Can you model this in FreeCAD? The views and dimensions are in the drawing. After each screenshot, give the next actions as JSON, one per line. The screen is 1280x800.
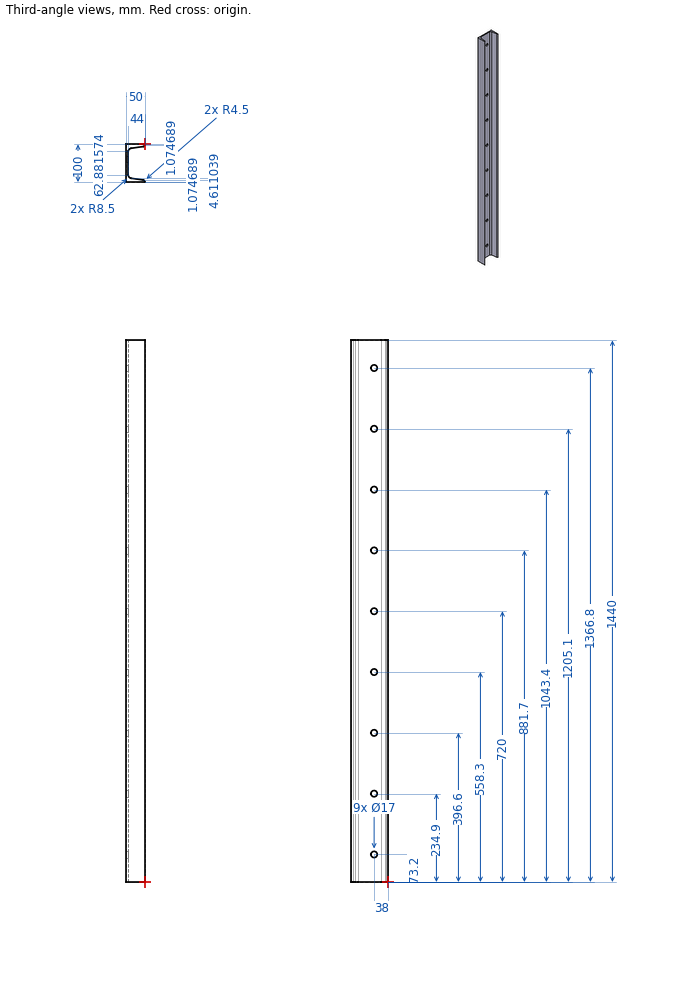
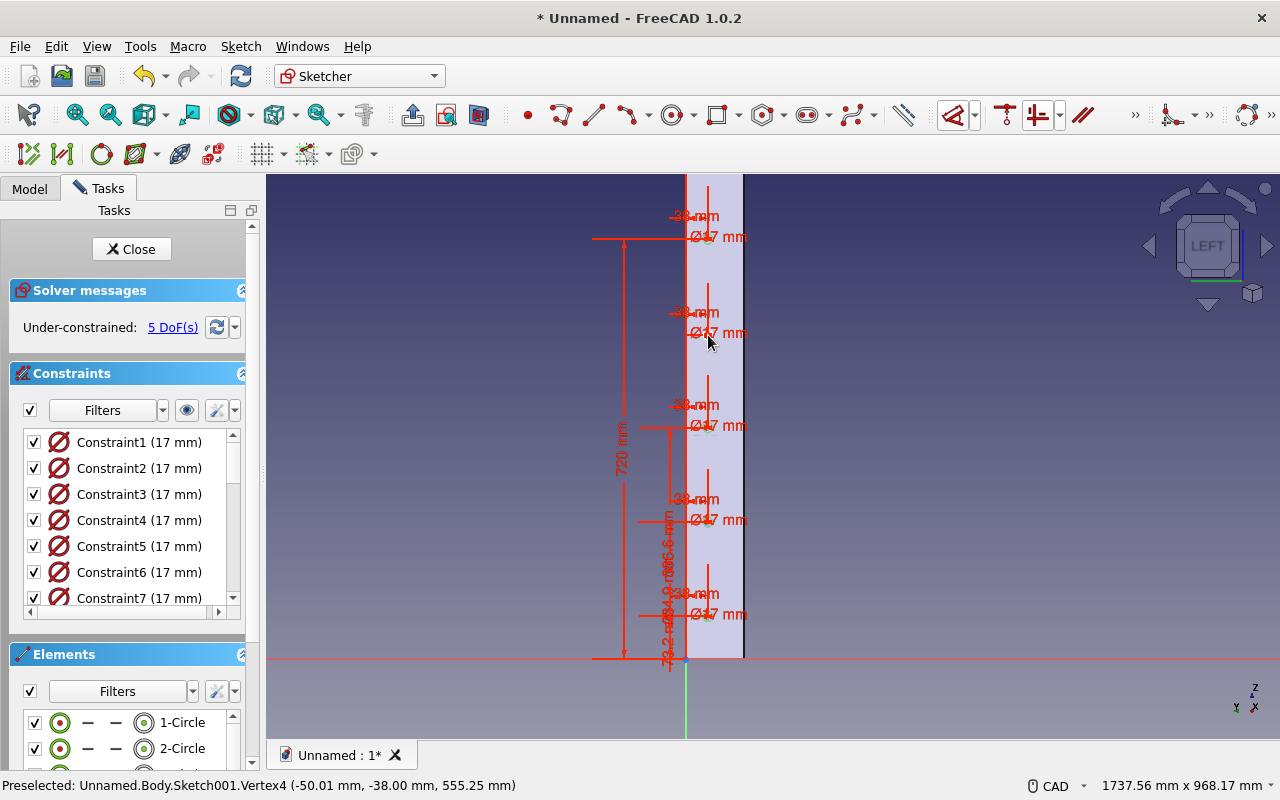
{"action": "left_click", "coordinate": [974, 116]}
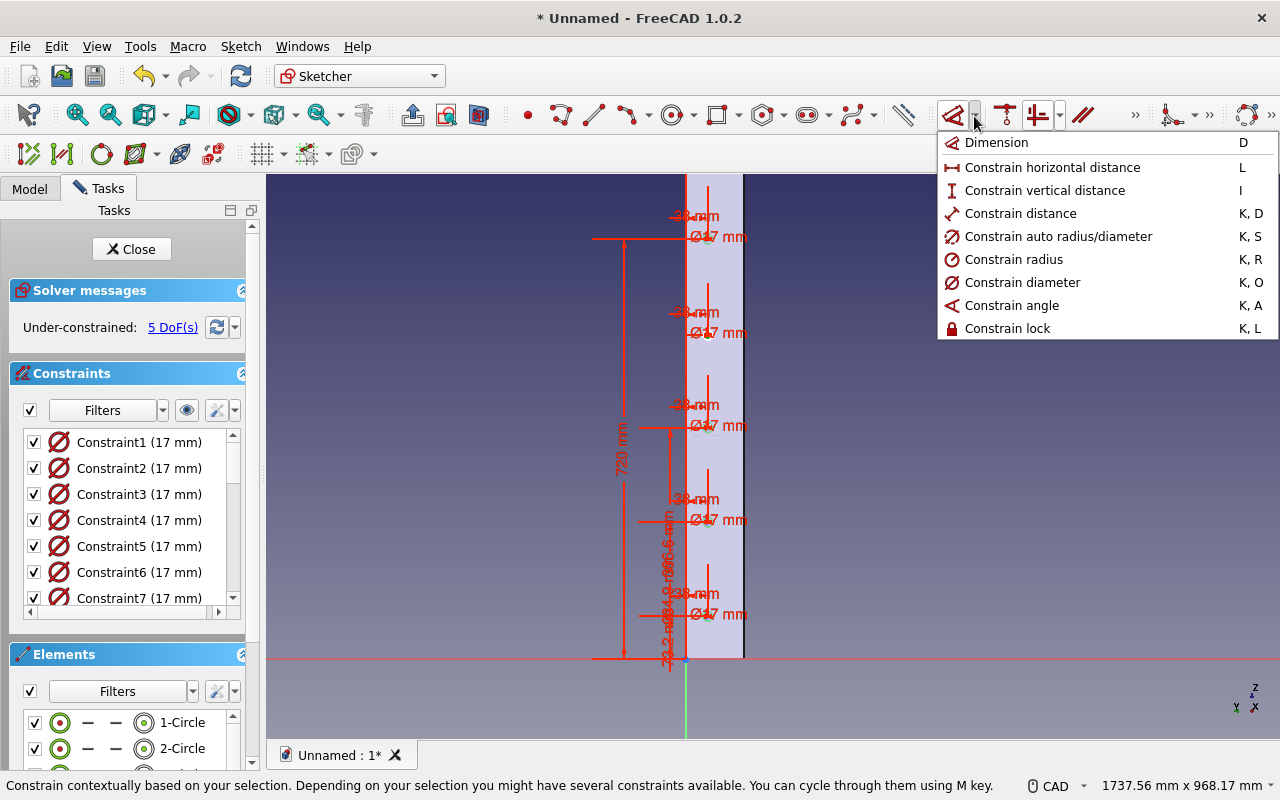
{"action": "left_click", "coordinate": [1108, 190]}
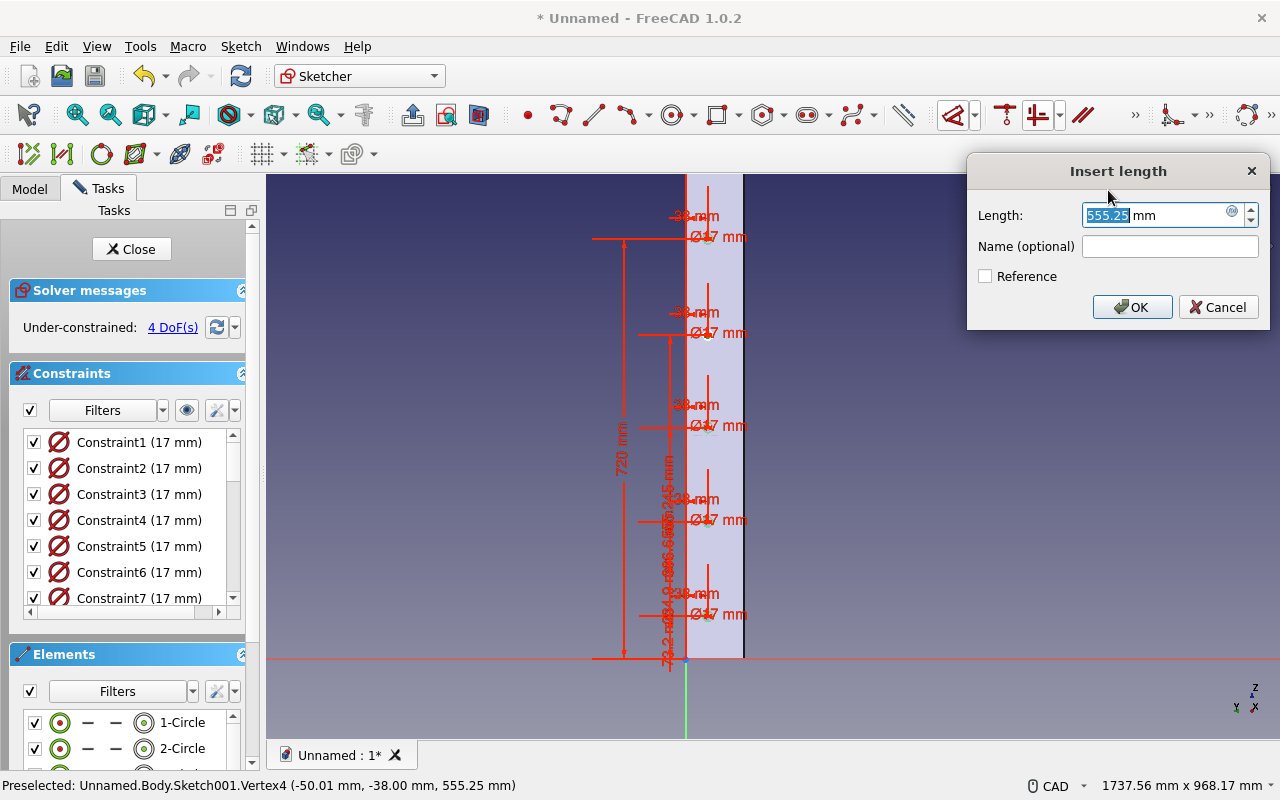
{"action": "type", "text": "558.3"}
{"action": "key", "text": "Return"}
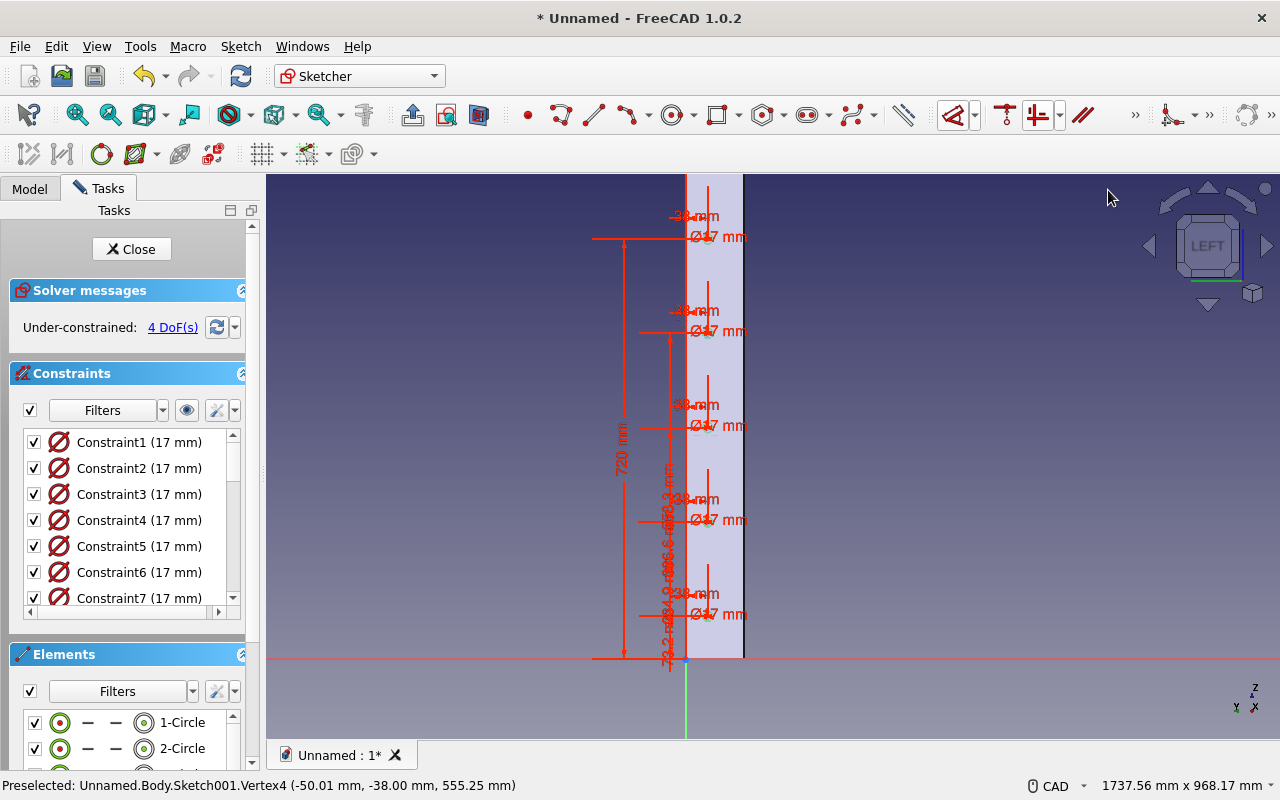
{"action": "scroll", "coordinate": [709, 619], "scroll_direction": "down", "scroll_amount": 4}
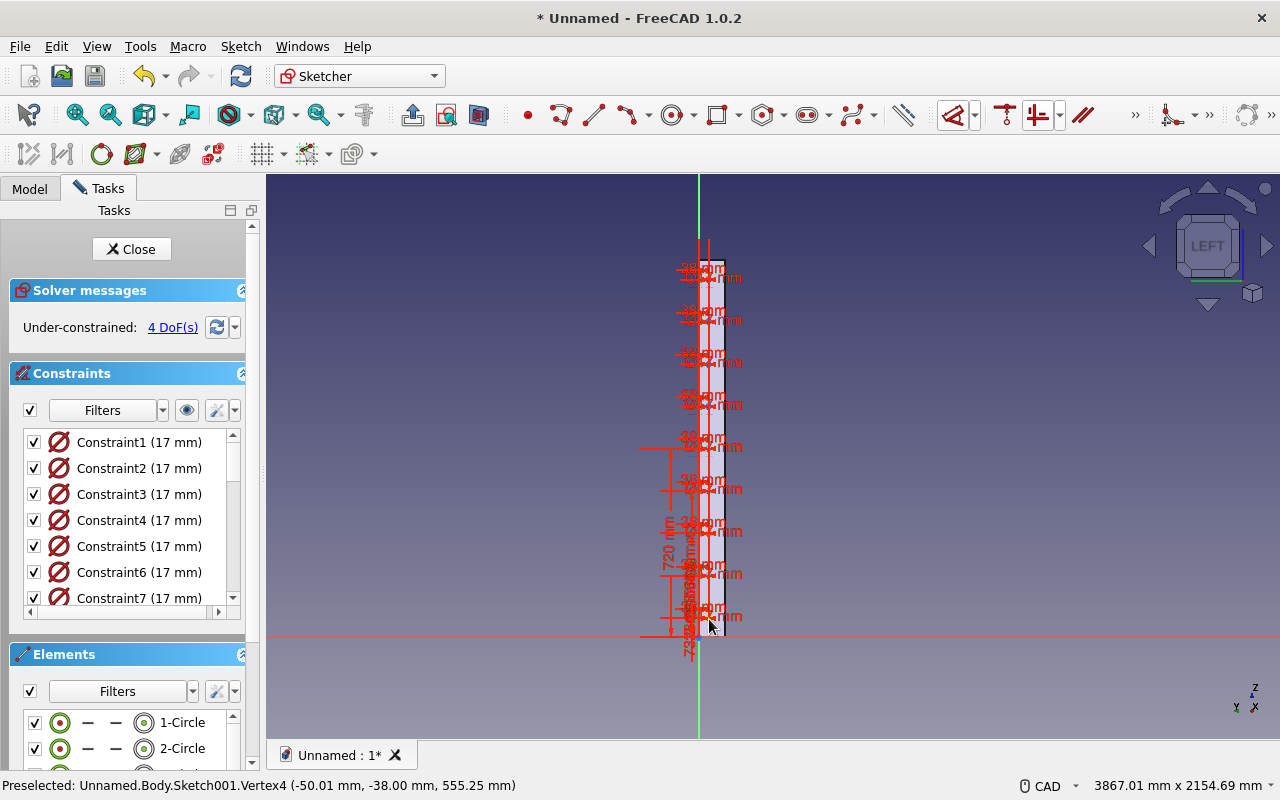
{"action": "left_click", "coordinate": [709, 407]}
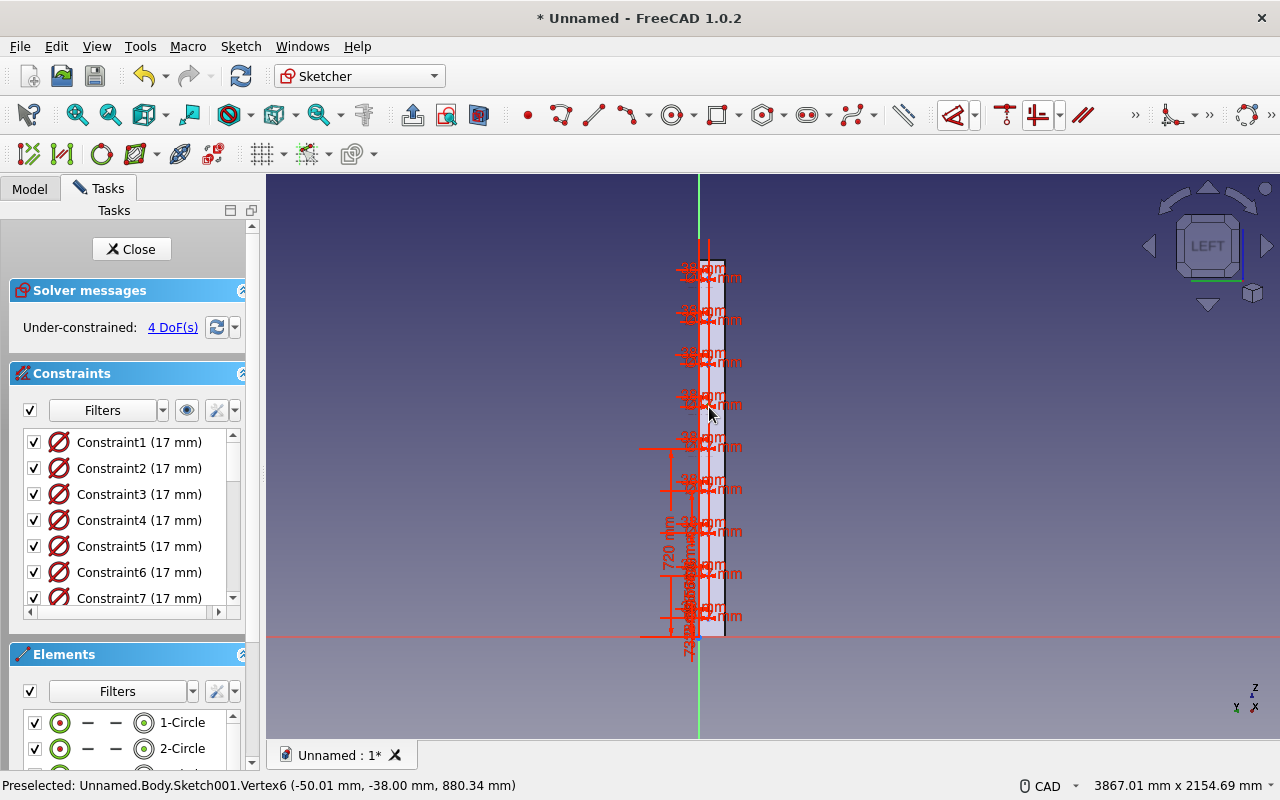
{"action": "key", "text": "i"}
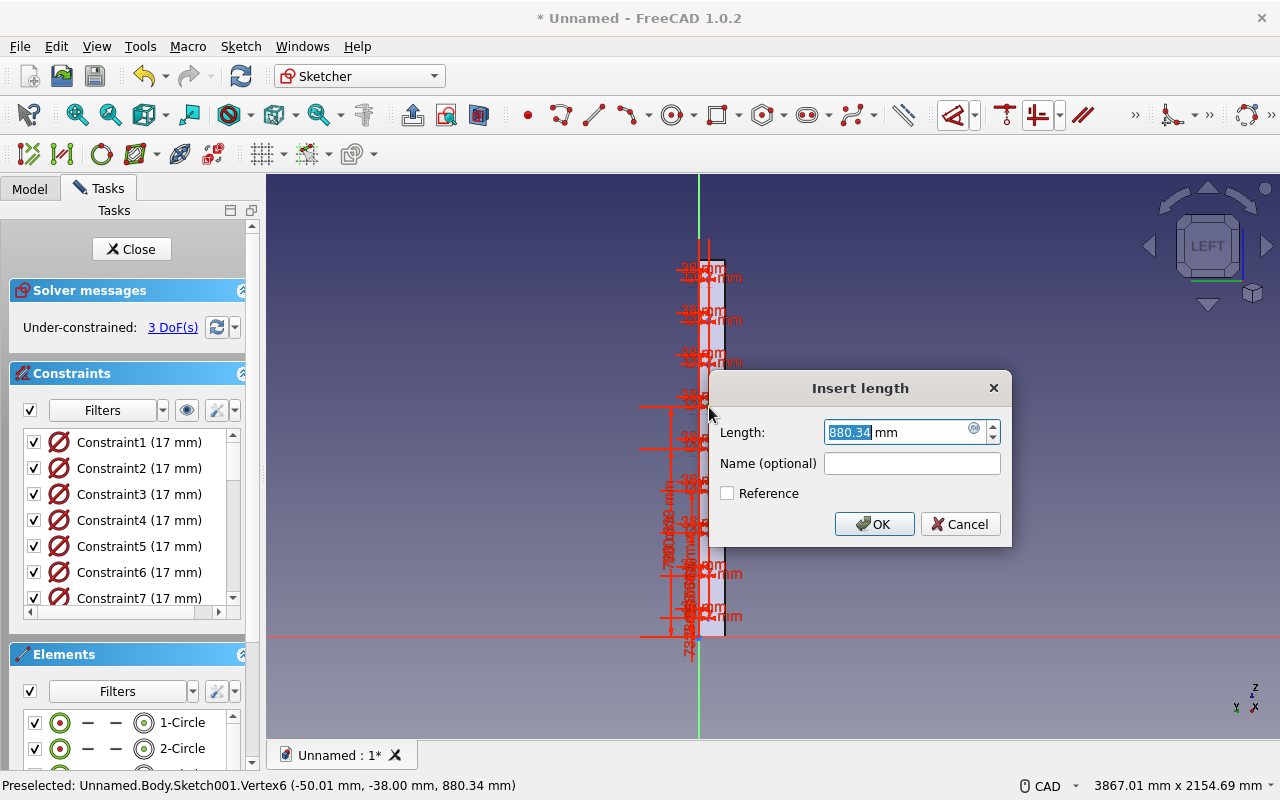
{"action": "type", "text": "881.7"}
{"action": "key", "text": "Return"}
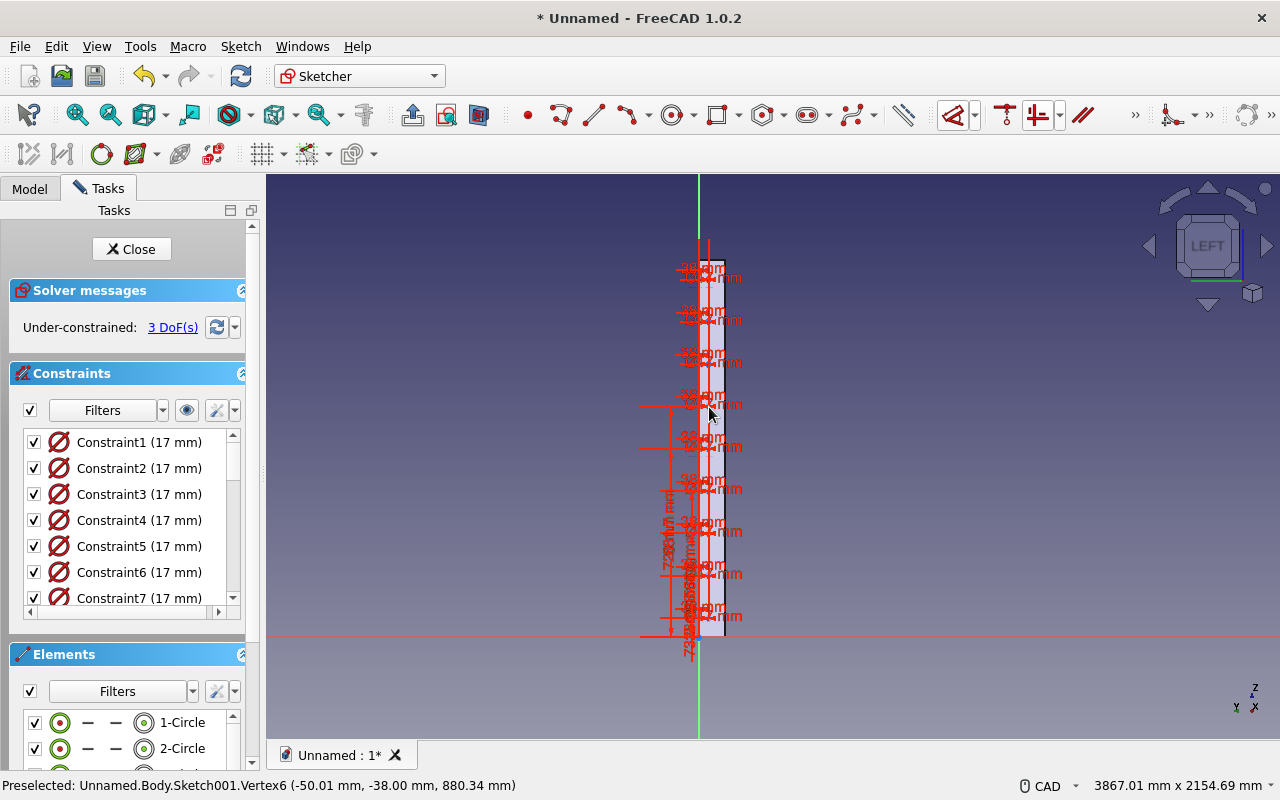
{"action": "left_click", "coordinate": [709, 364]}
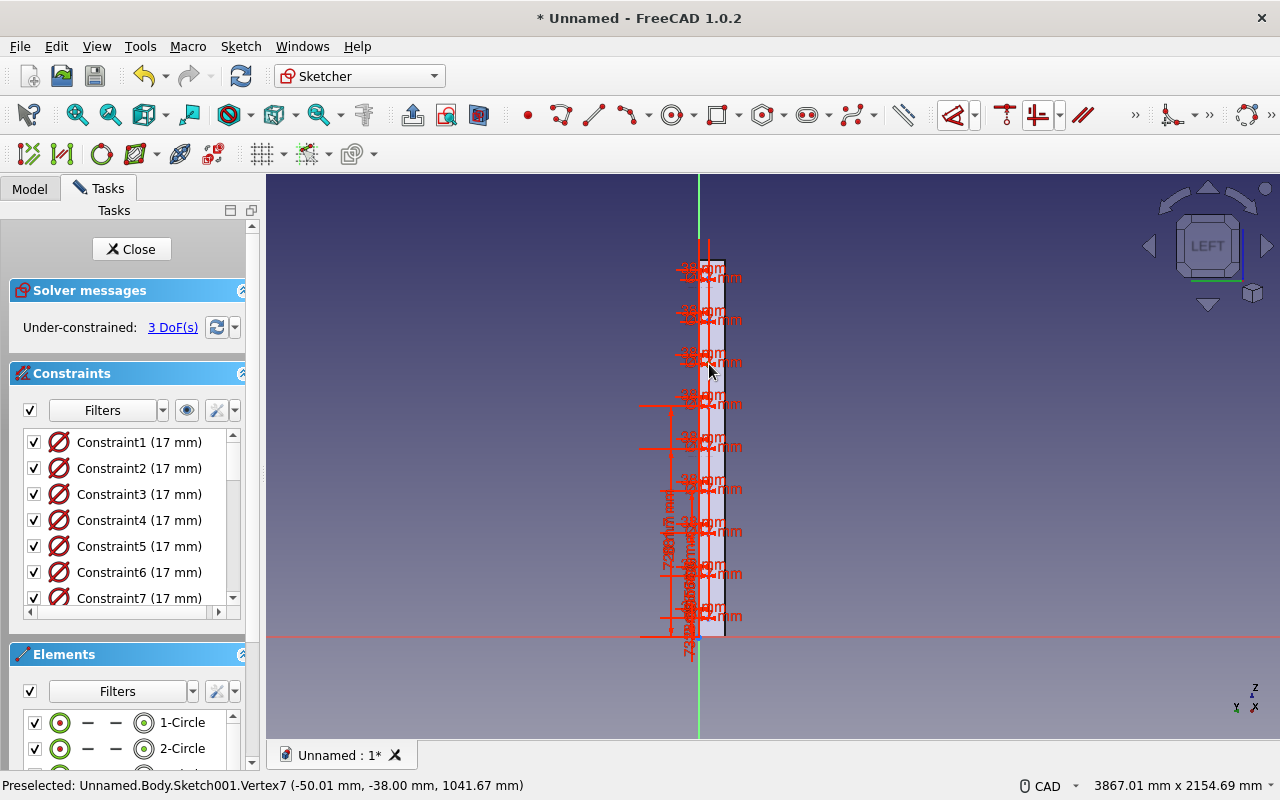
{"action": "key", "text": "i"}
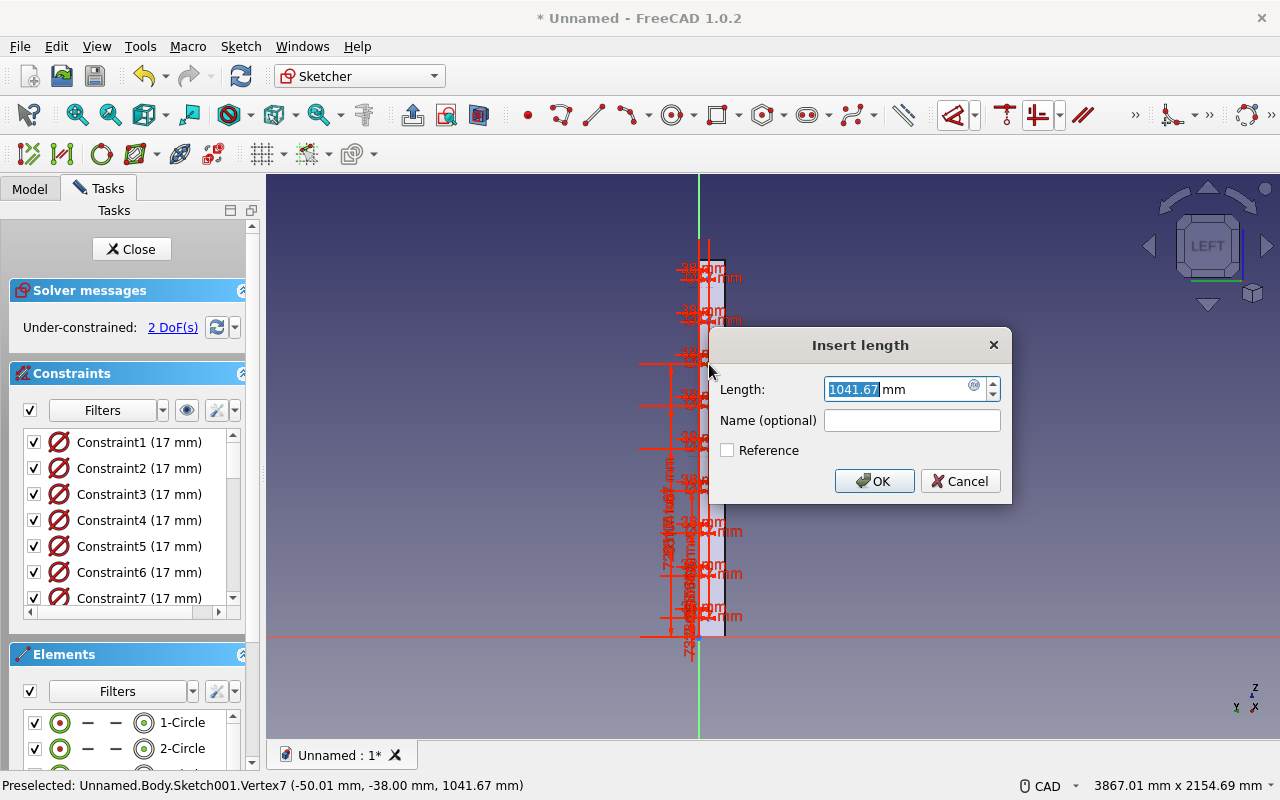
{"action": "type", "text": "1043.4"}
{"action": "key", "text": "Return"}